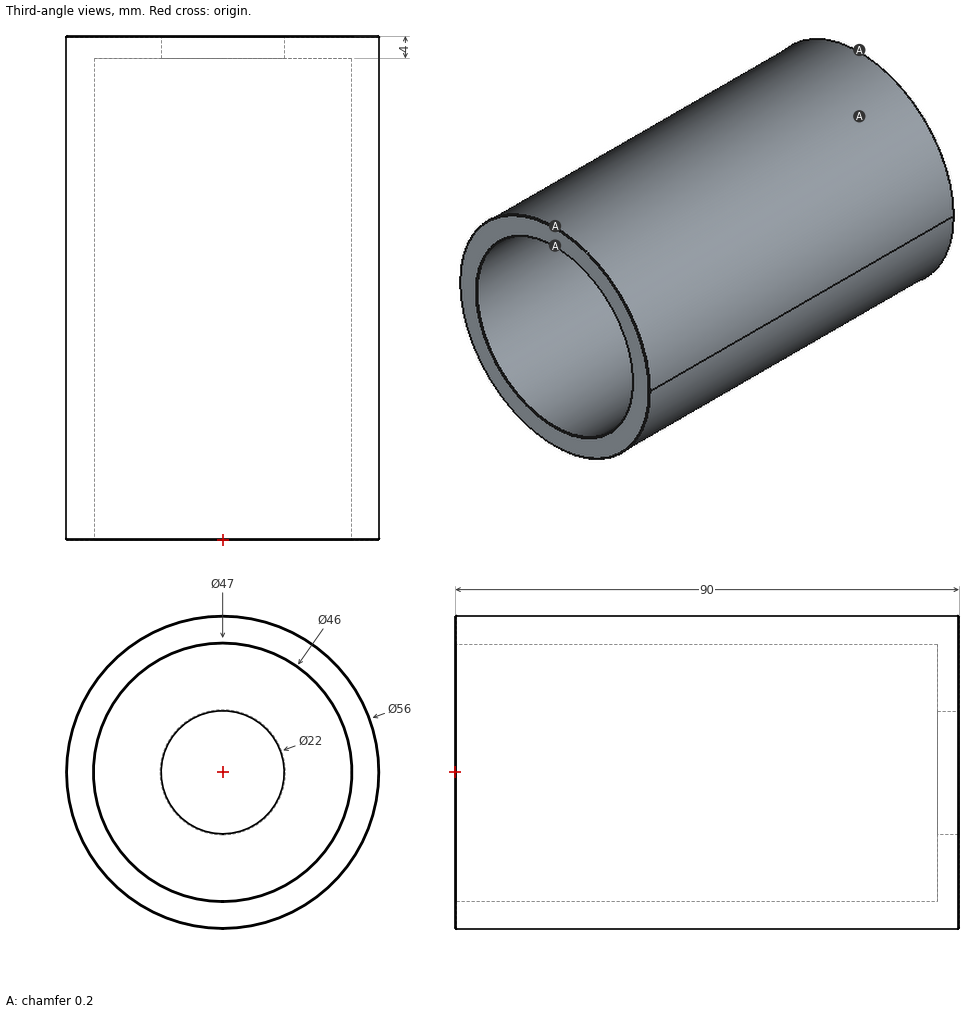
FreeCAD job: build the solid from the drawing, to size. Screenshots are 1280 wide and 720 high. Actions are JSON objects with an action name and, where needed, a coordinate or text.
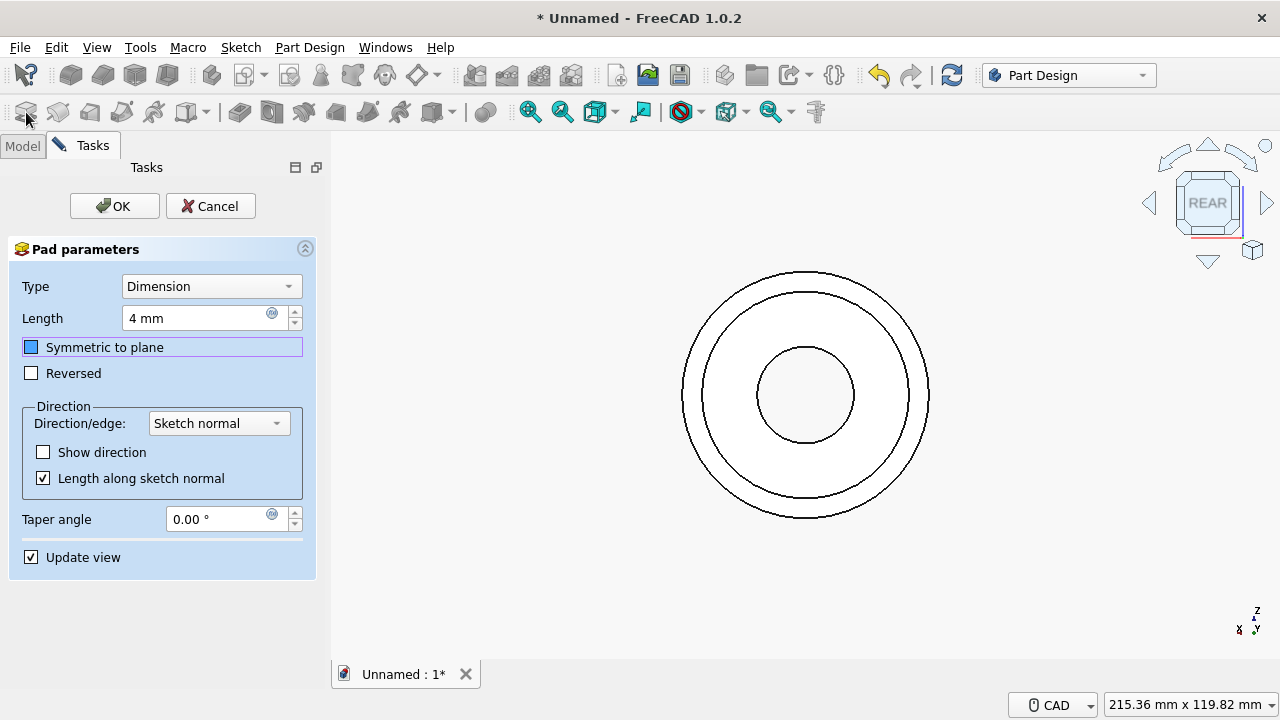
{"action": "left_click", "coordinate": [30, 373]}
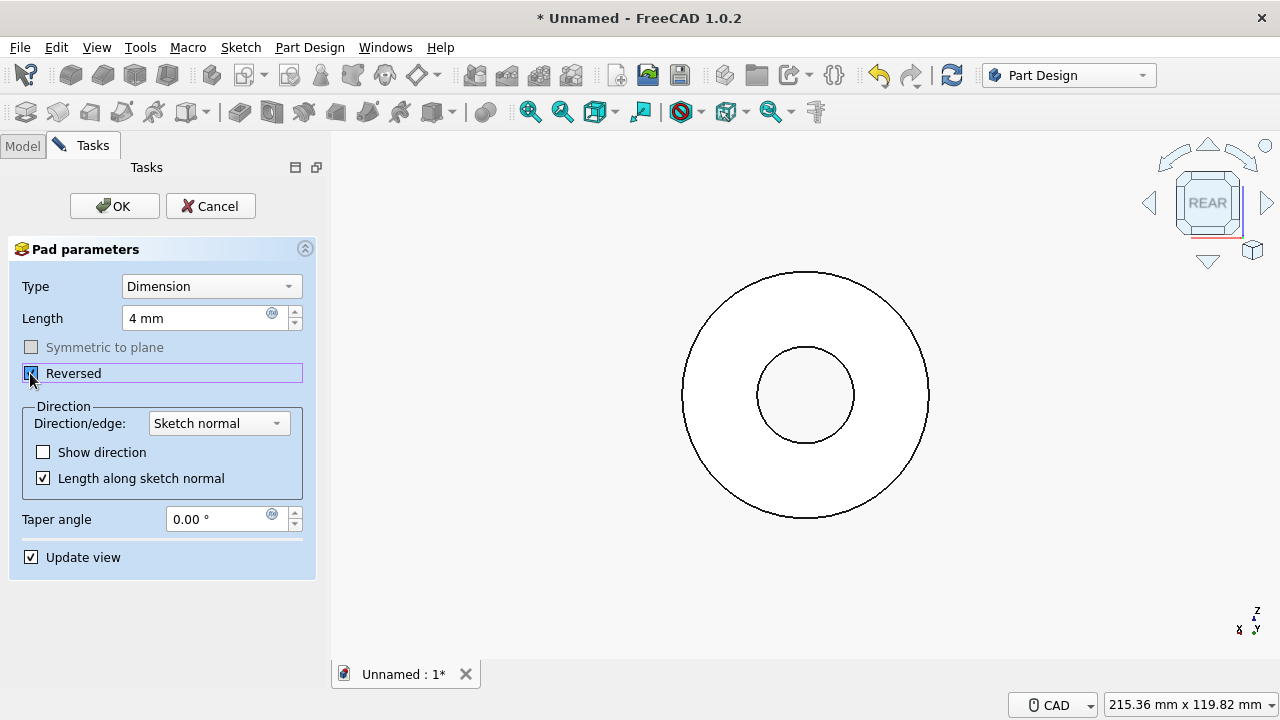
{"action": "left_click", "coordinate": [115, 206]}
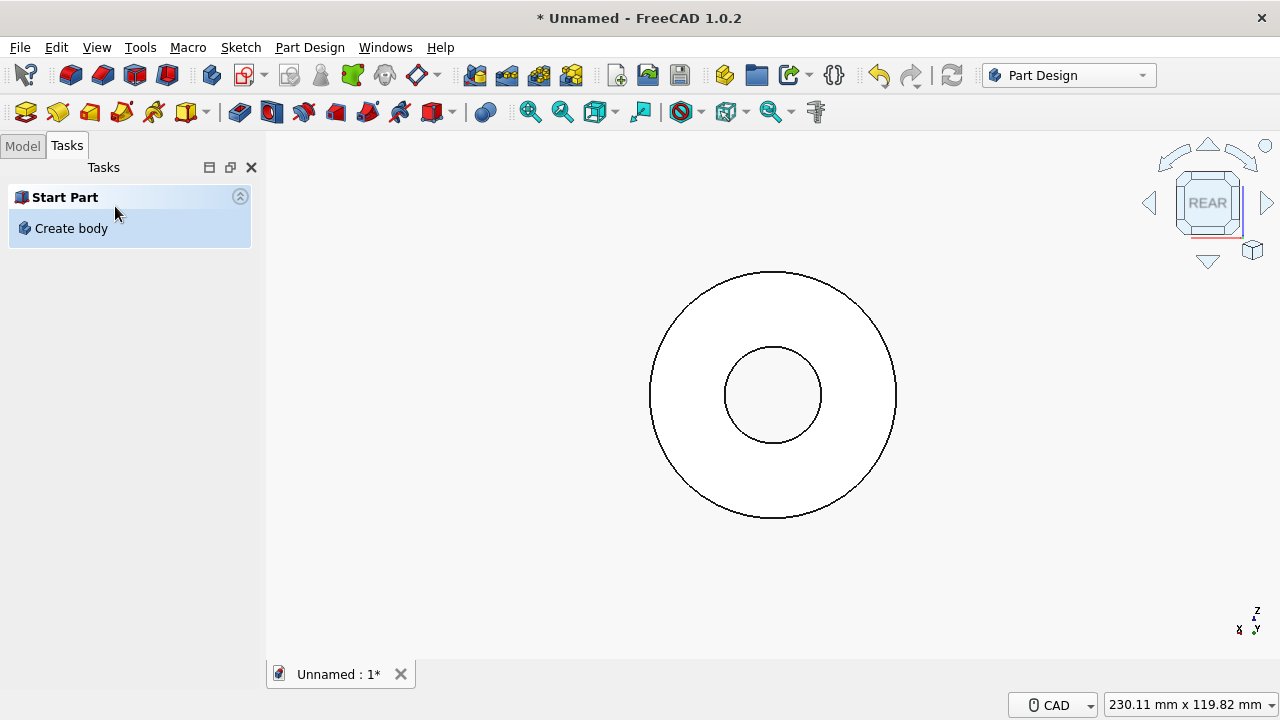
{"action": "left_click", "coordinate": [812, 366]}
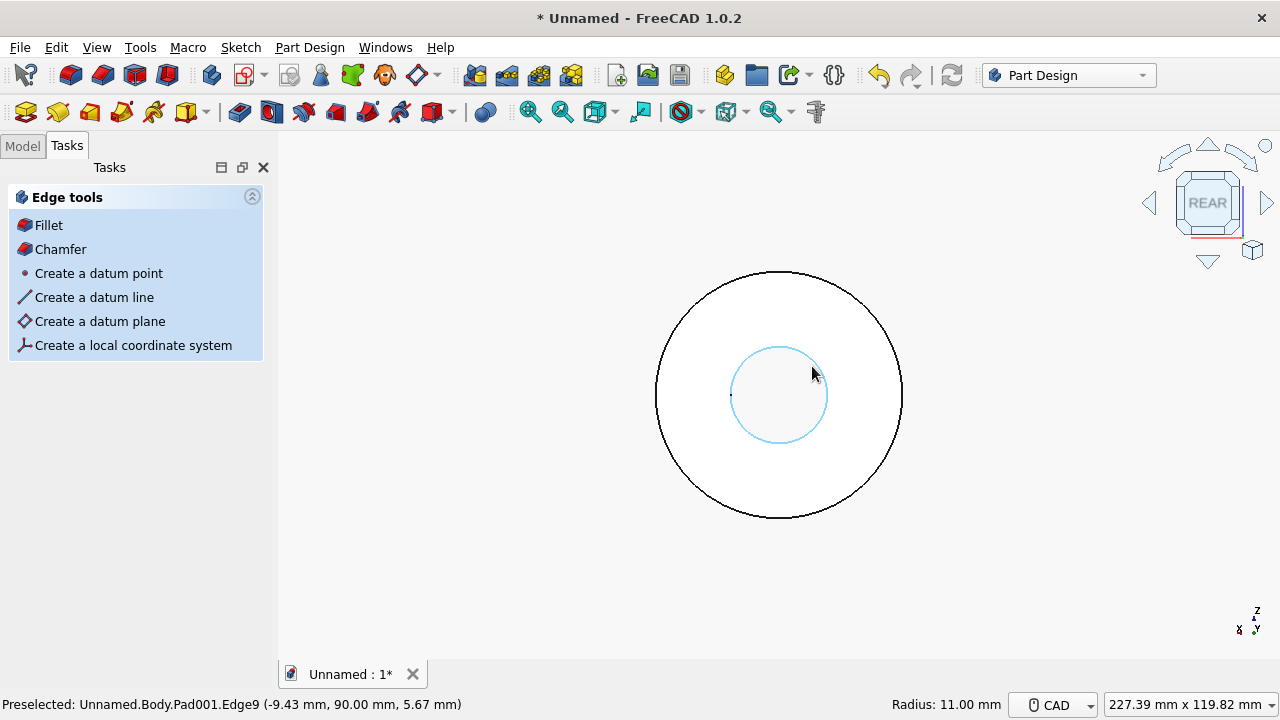
{"action": "left_click", "coordinate": [902, 394], "text": "ctrl"}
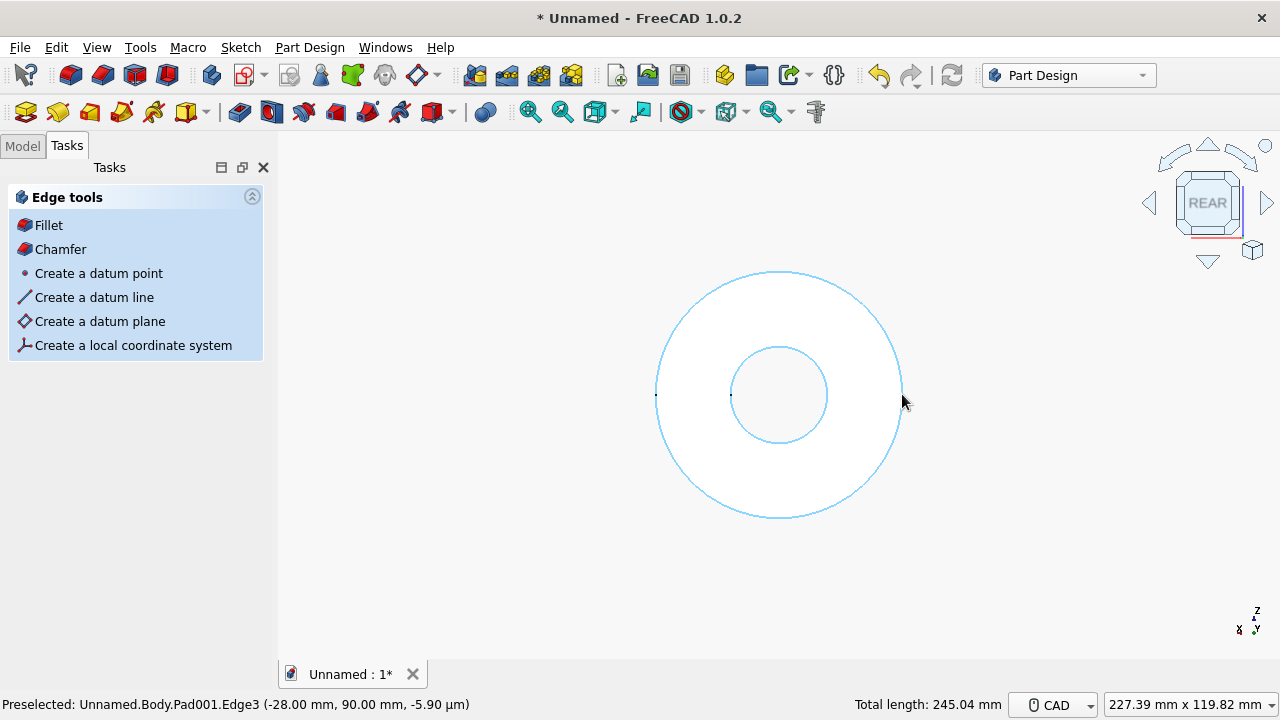
{"action": "key", "text": "0"}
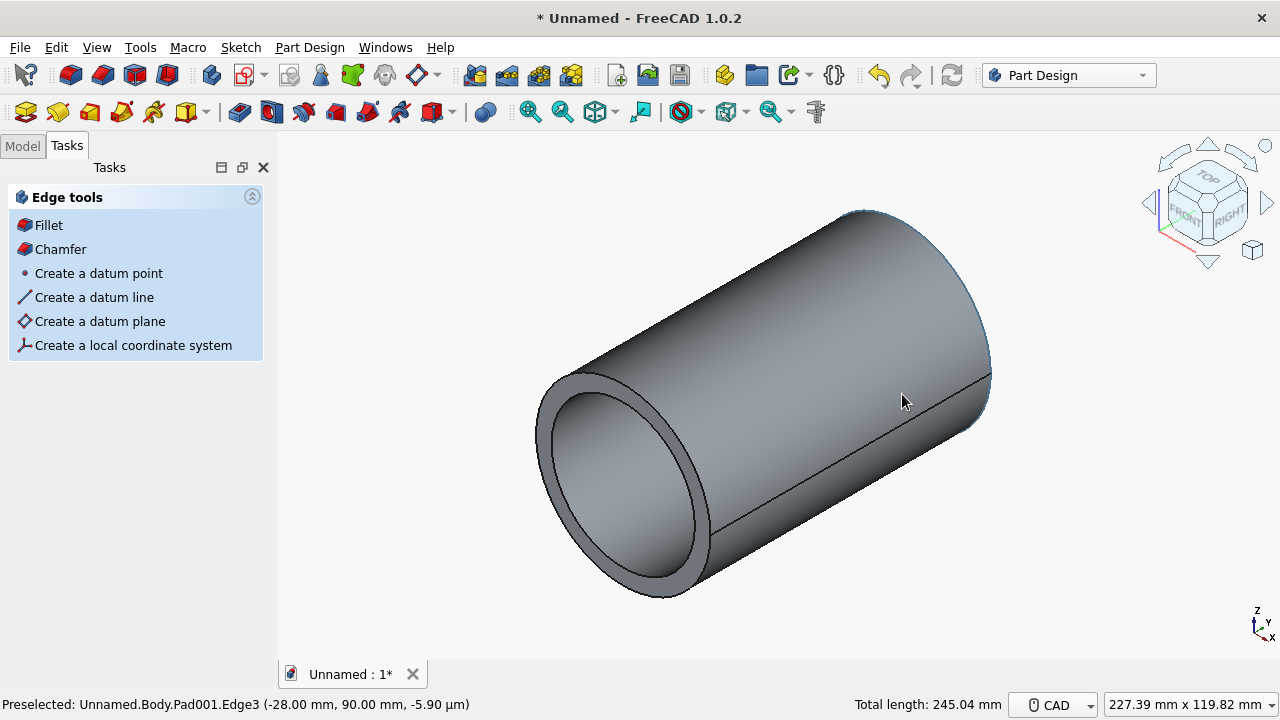
{"action": "left_click", "coordinate": [596, 373], "text": "ctrl"}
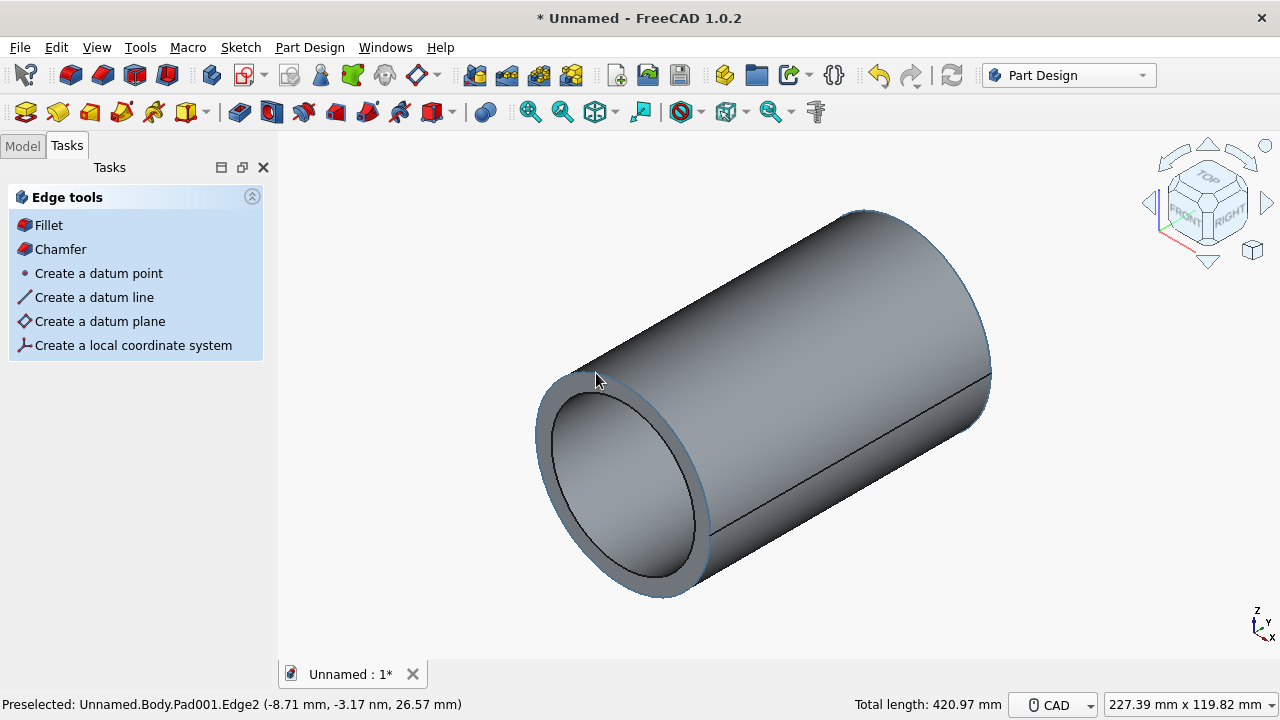
{"action": "left_click", "coordinate": [552, 443], "text": "ctrl"}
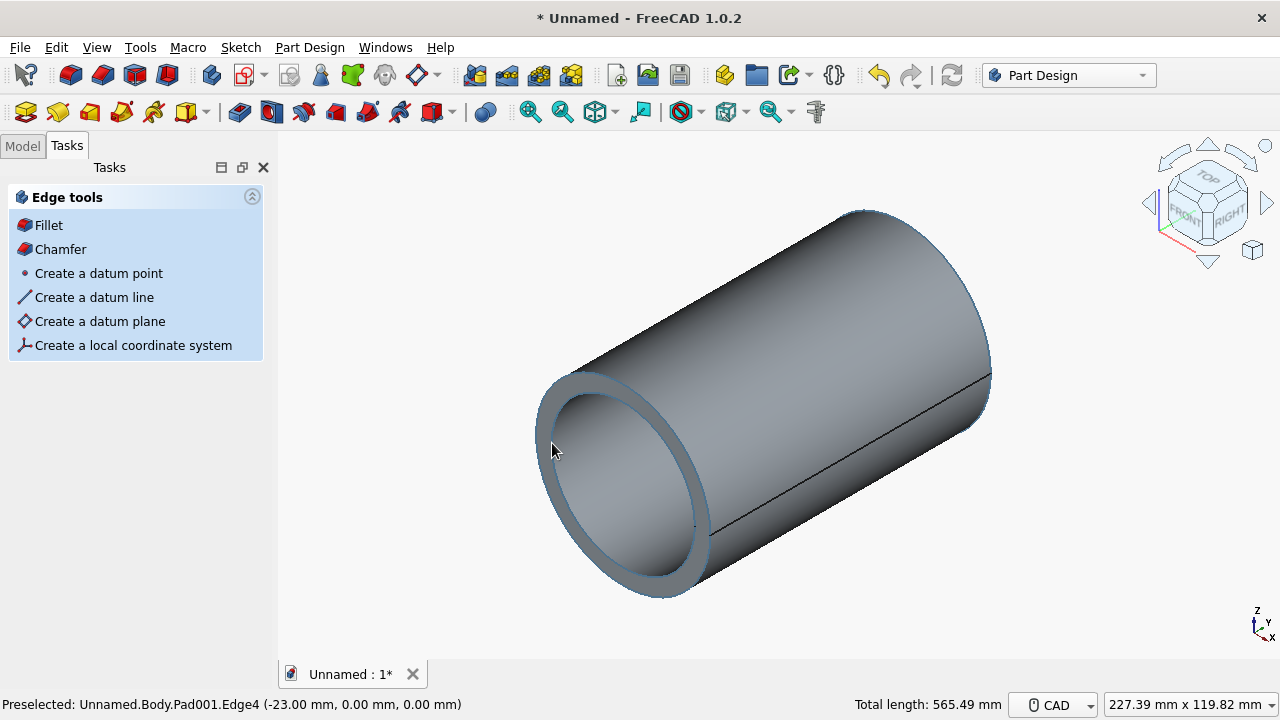
{"action": "left_click", "coordinate": [104, 76]}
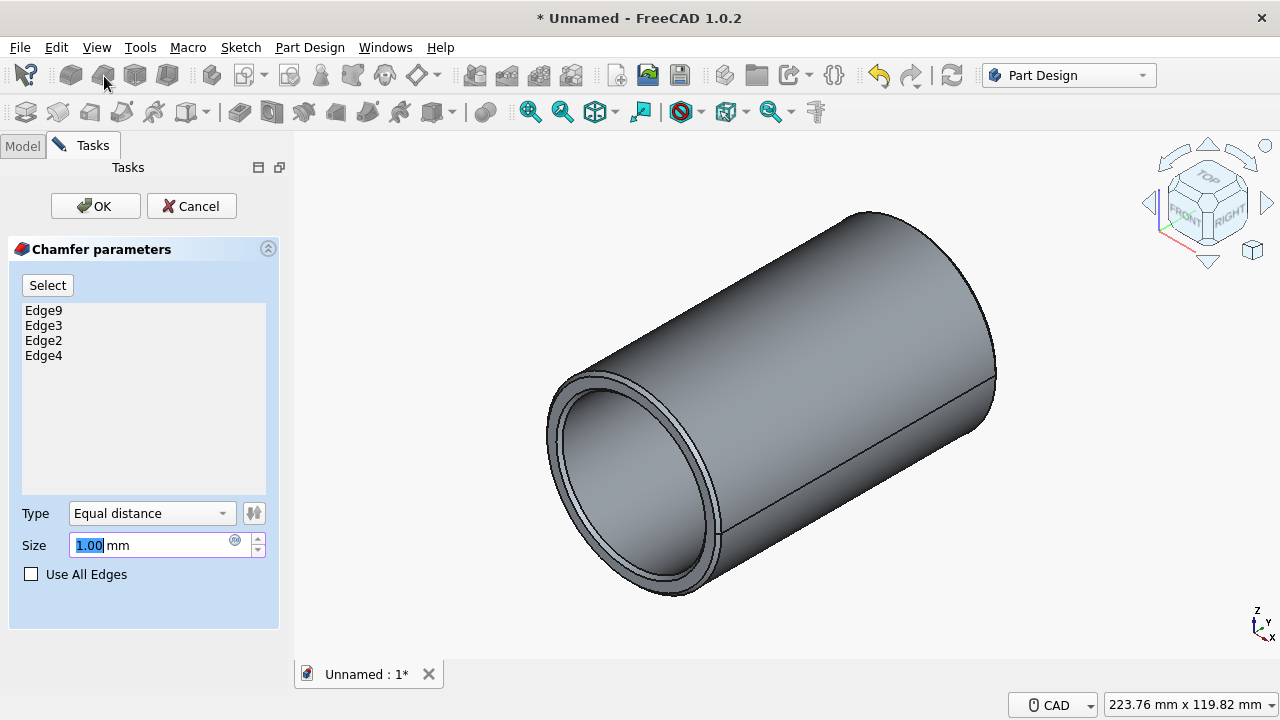
{"action": "type", "text": "0.2"}
{"action": "key", "text": "Tab"}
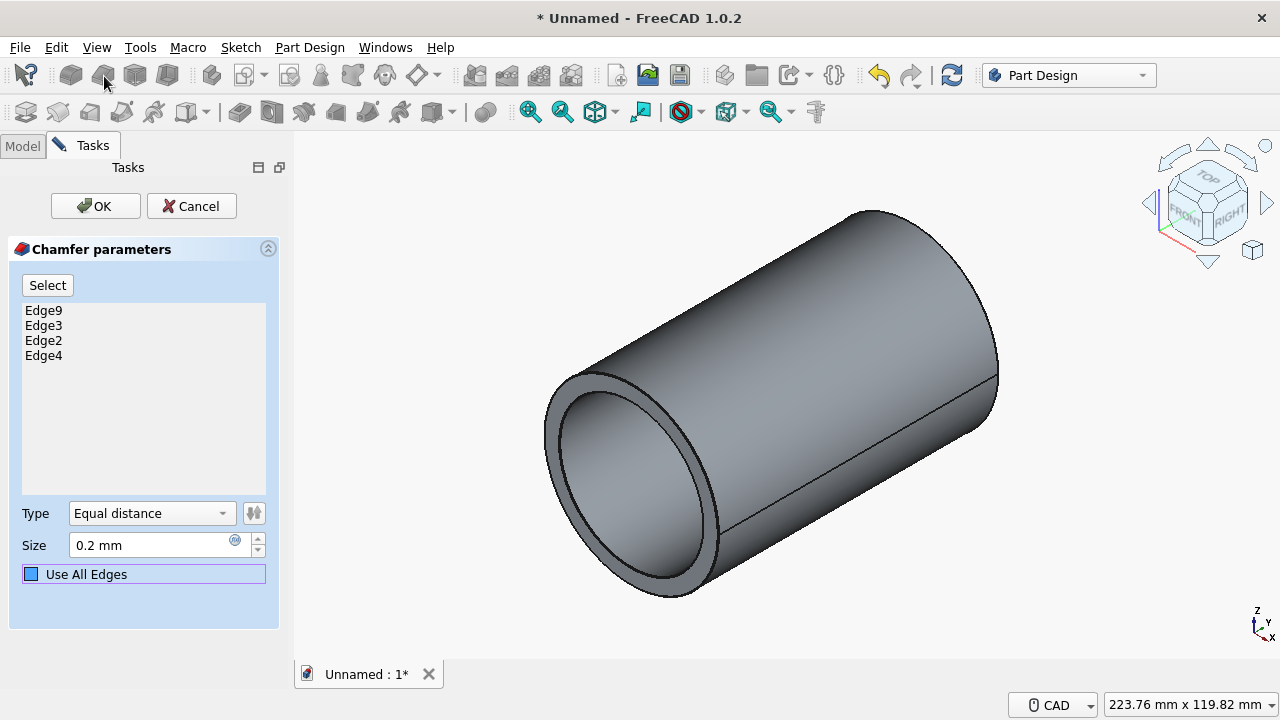
{"action": "left_click", "coordinate": [96, 206]}